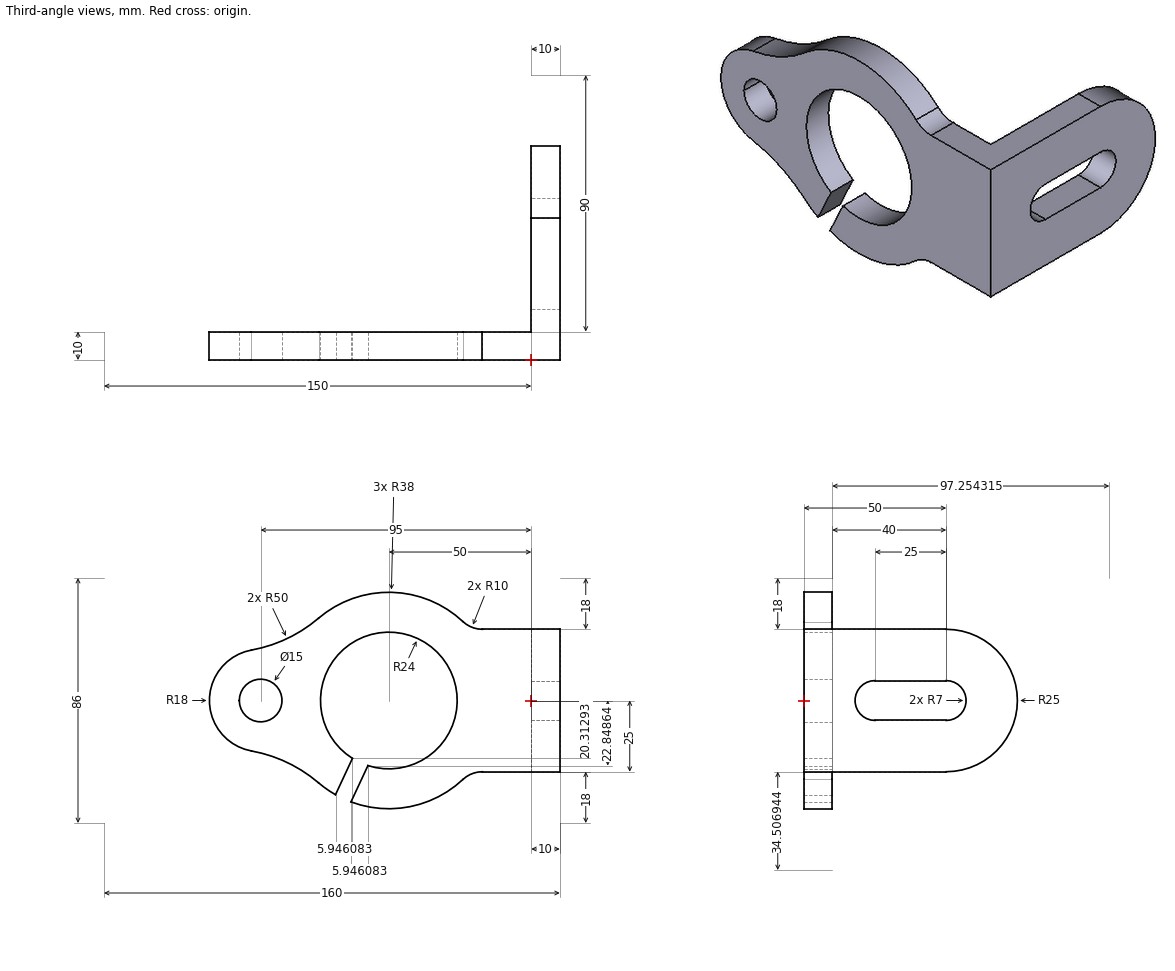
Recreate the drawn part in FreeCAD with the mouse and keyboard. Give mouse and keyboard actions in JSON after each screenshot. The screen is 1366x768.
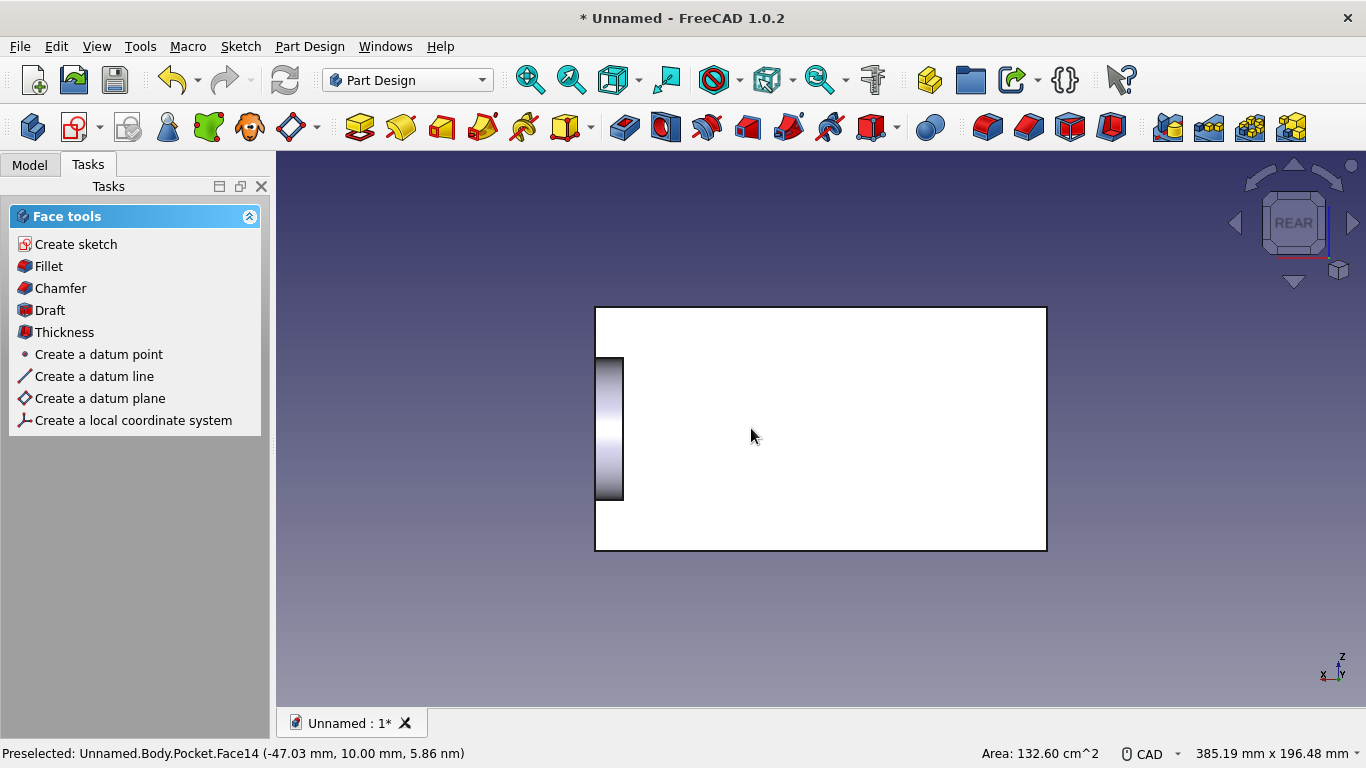
{"action": "left_click", "coordinate": [74, 128]}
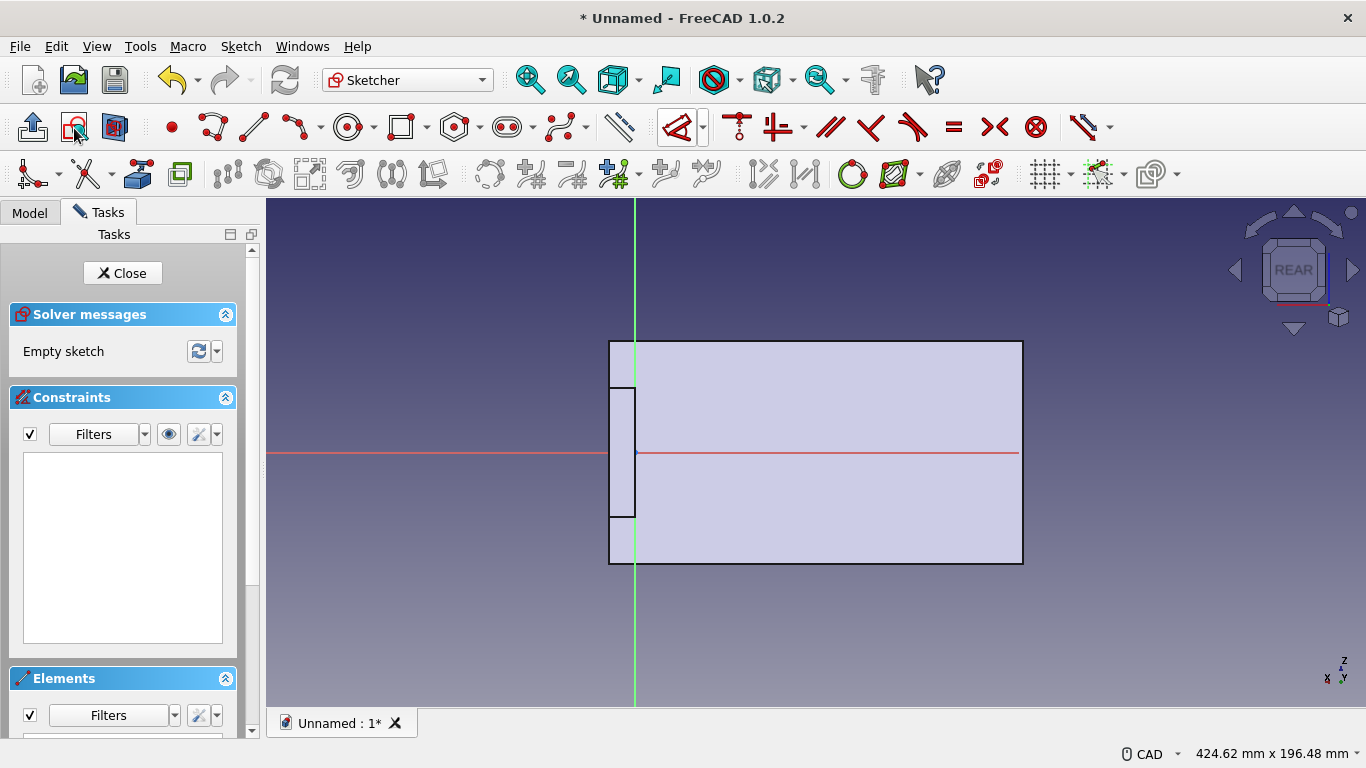
{"action": "key", "text": "q s"}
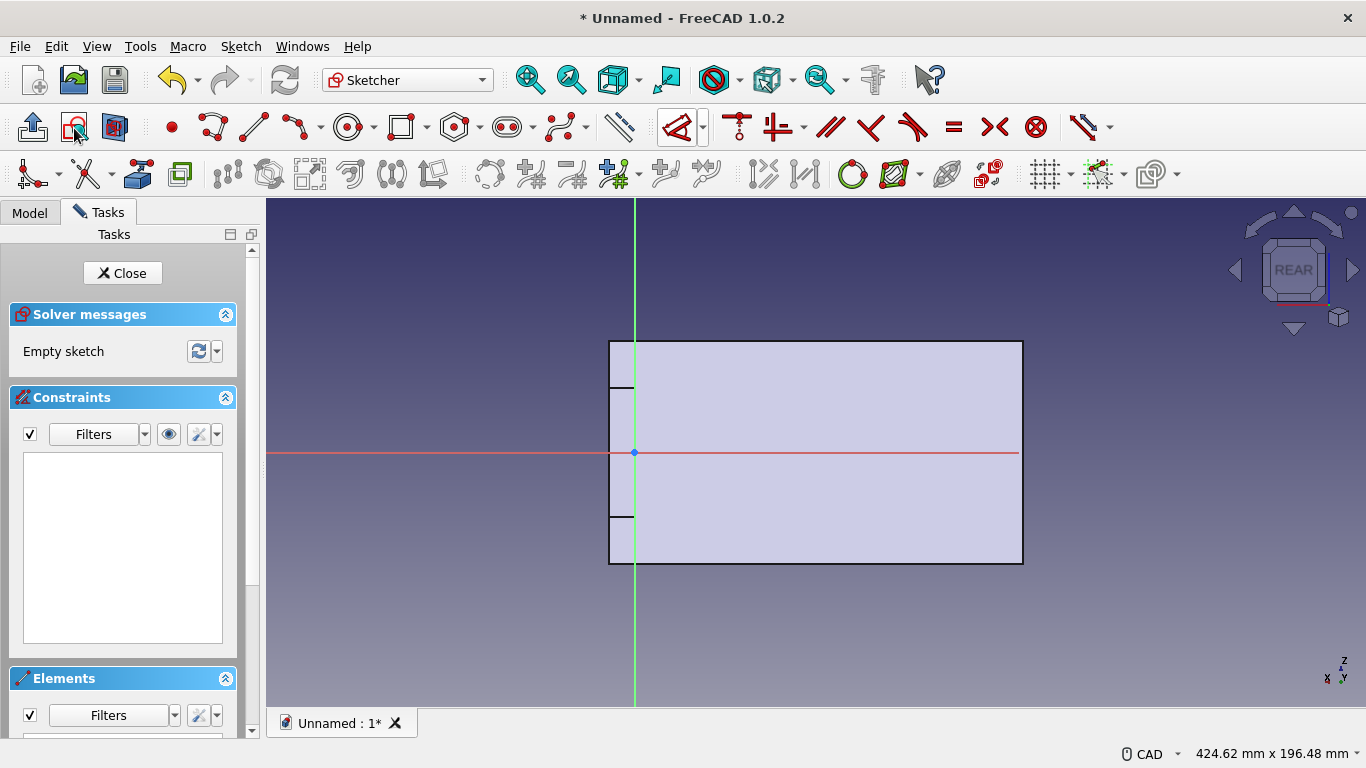
{"action": "scroll", "coordinate": [955, 453], "scroll_direction": "up", "scroll_amount": 2}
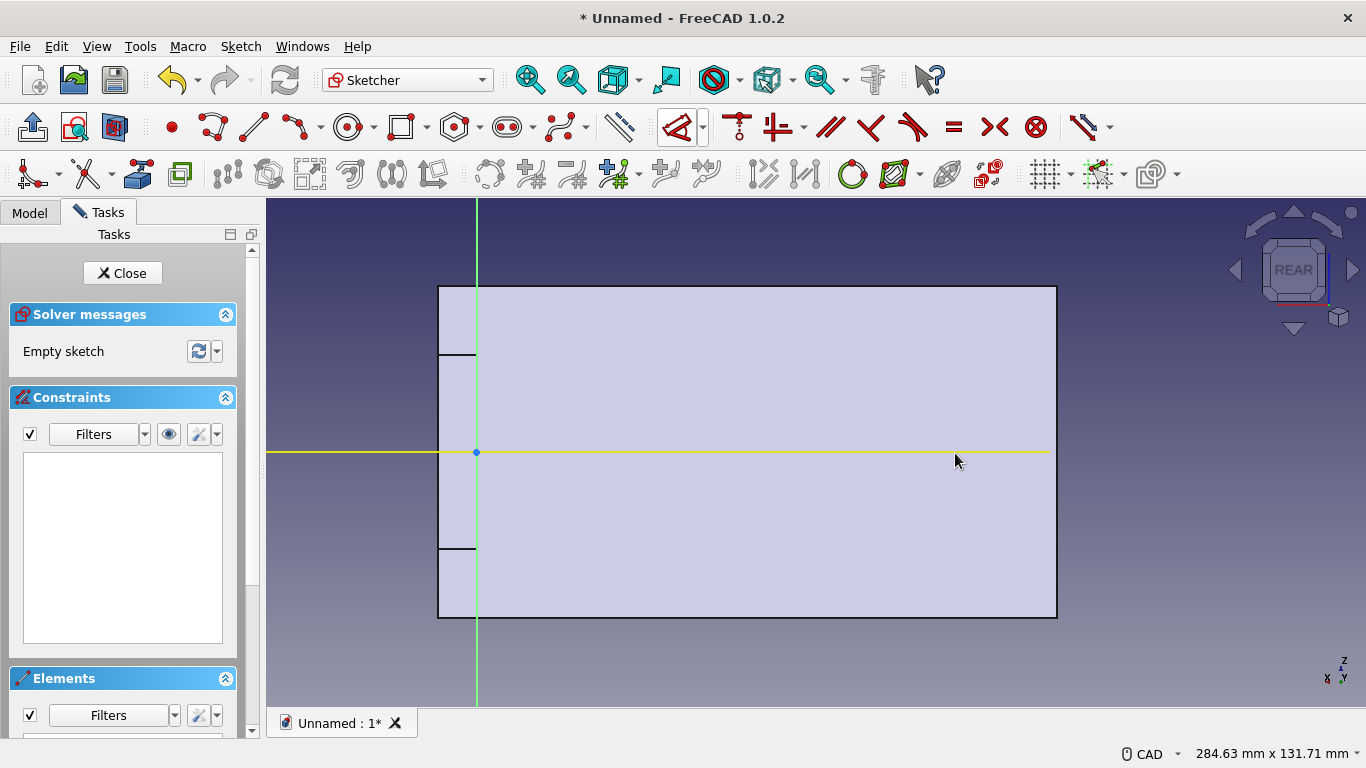
{"action": "key", "text": "g l"}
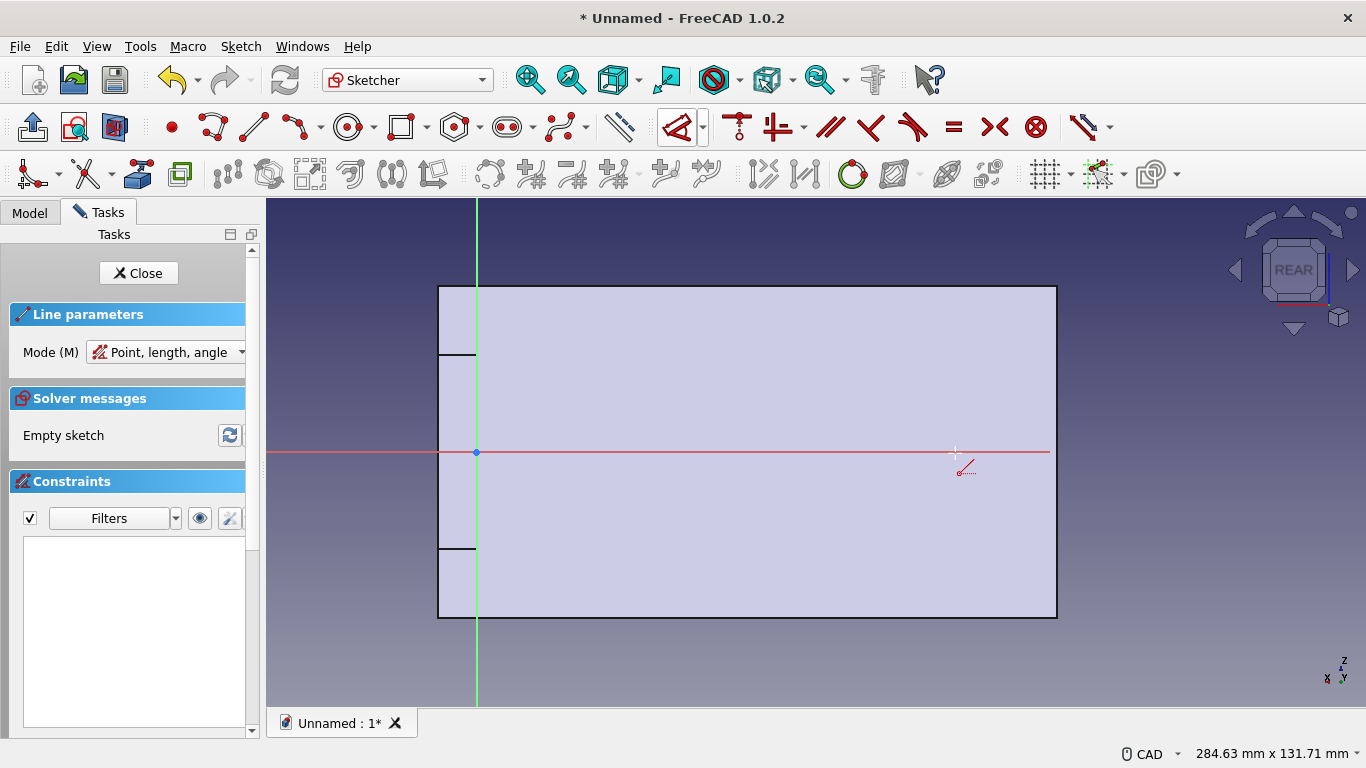
{"action": "left_click", "coordinate": [742, 580]}
{"action": "left_click", "coordinate": [719, 531]}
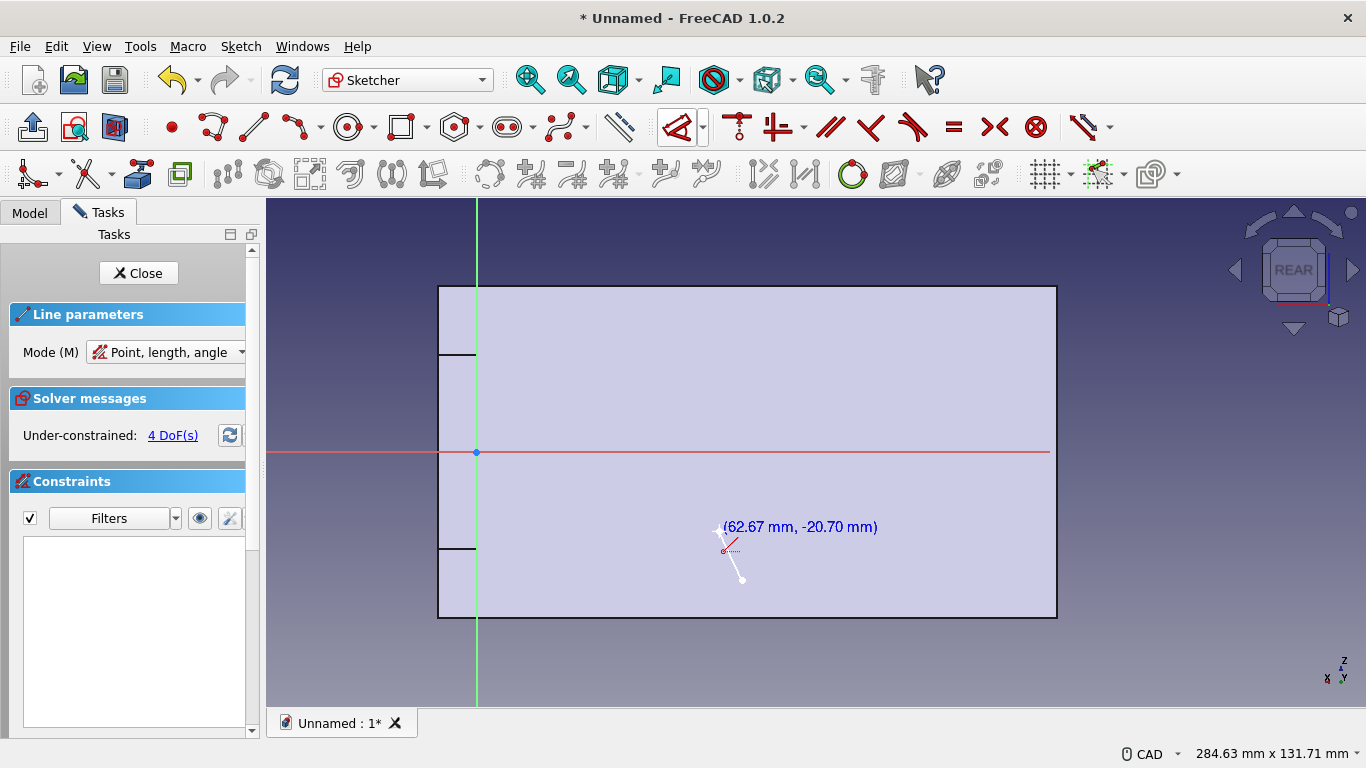
{"action": "left_click", "coordinate": [698, 540]}
{"action": "left_click", "coordinate": [721, 590]}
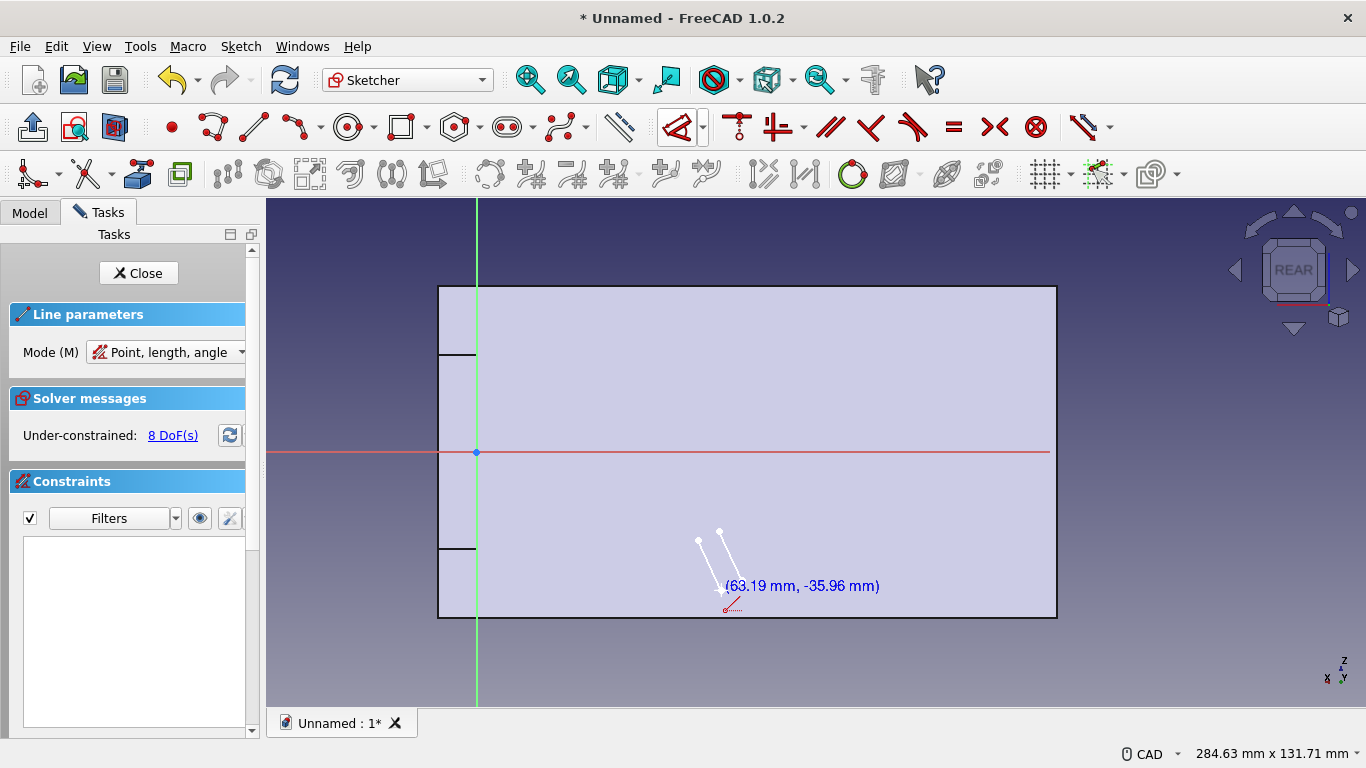
{"action": "left_click", "coordinate": [213, 128]}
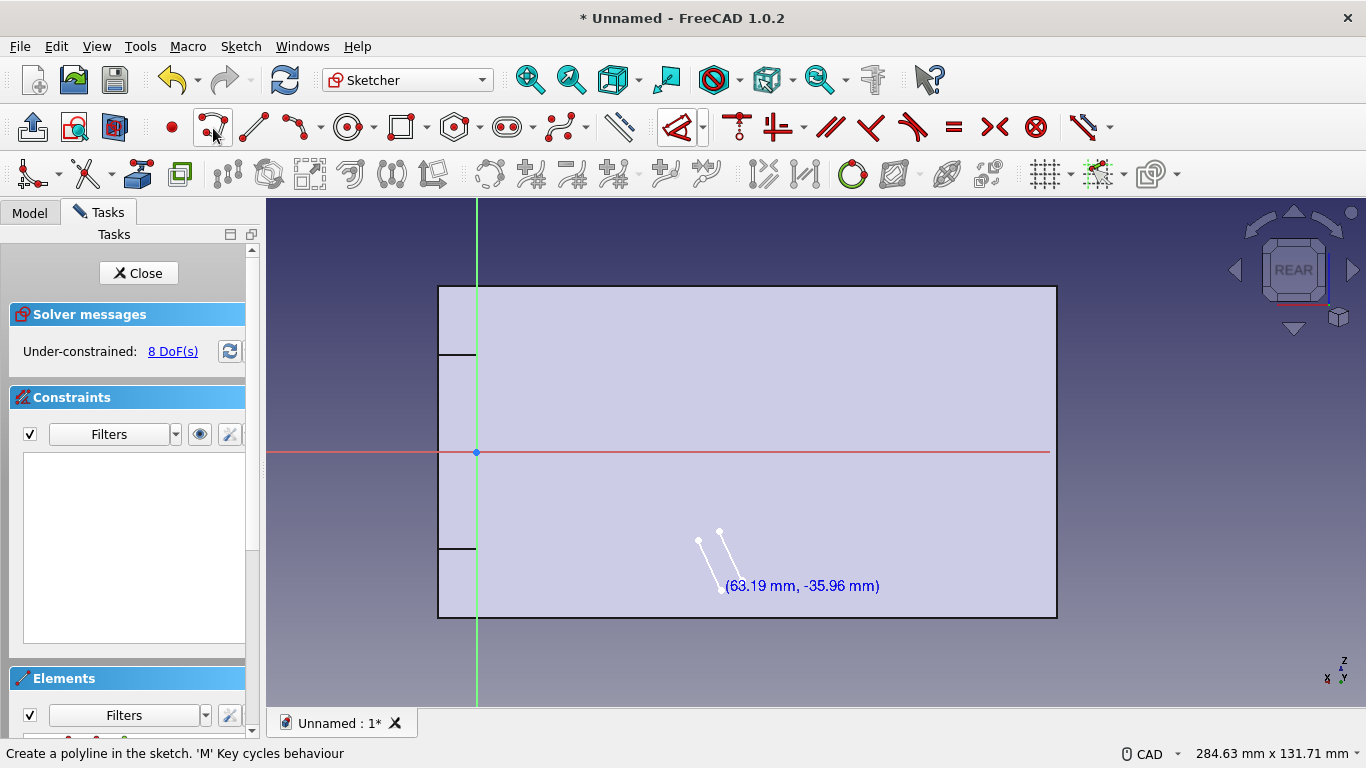
{"action": "left_click", "coordinate": [543, 549]}
{"action": "left_click", "coordinate": [438, 549]}
{"action": "left_click", "coordinate": [438, 618]}
{"action": "left_click", "coordinate": [1057, 618]}
{"action": "left_click", "coordinate": [1057, 286]}
{"action": "left_click", "coordinate": [438, 286]}
{"action": "left_click", "coordinate": [438, 355]}
{"action": "left_click", "coordinate": [543, 355]}
{"action": "right_click", "coordinate": [543, 355]}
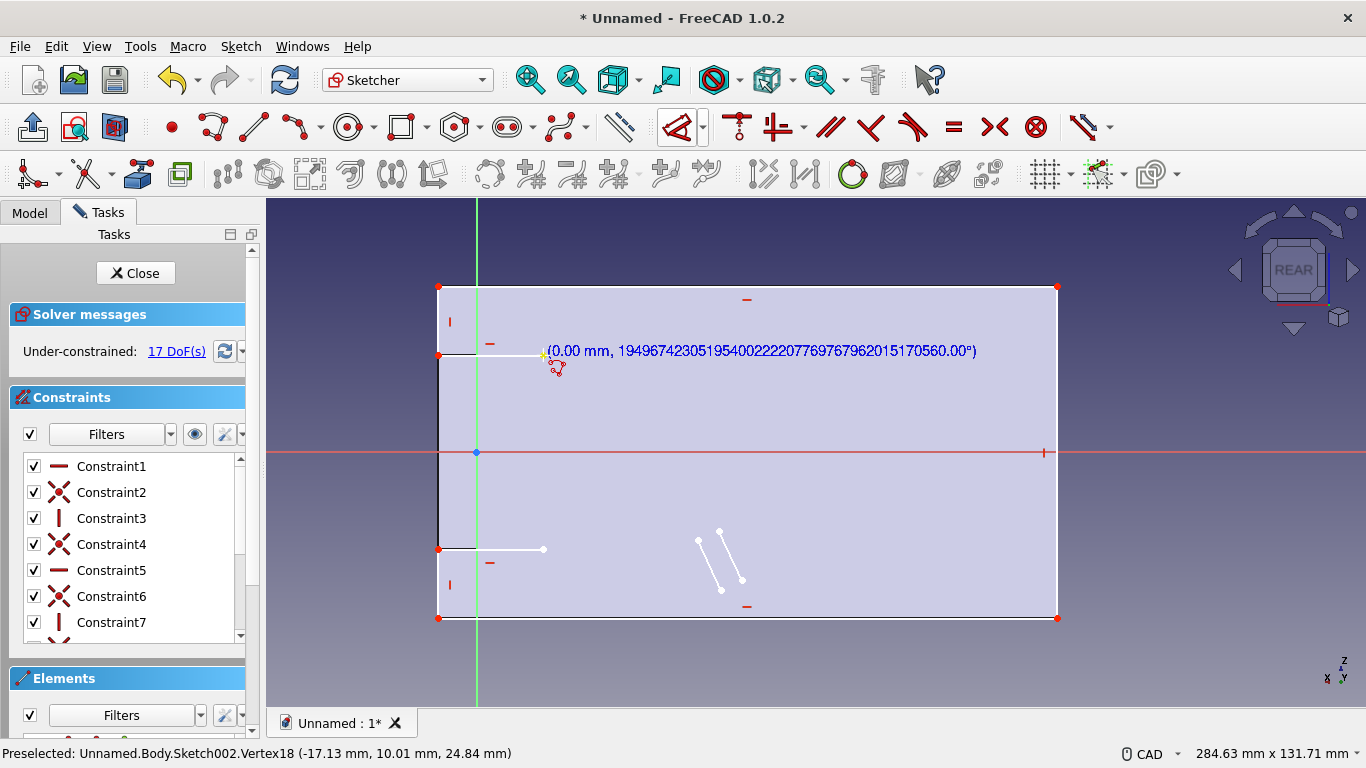
{"action": "key", "text": "g 3 a"}